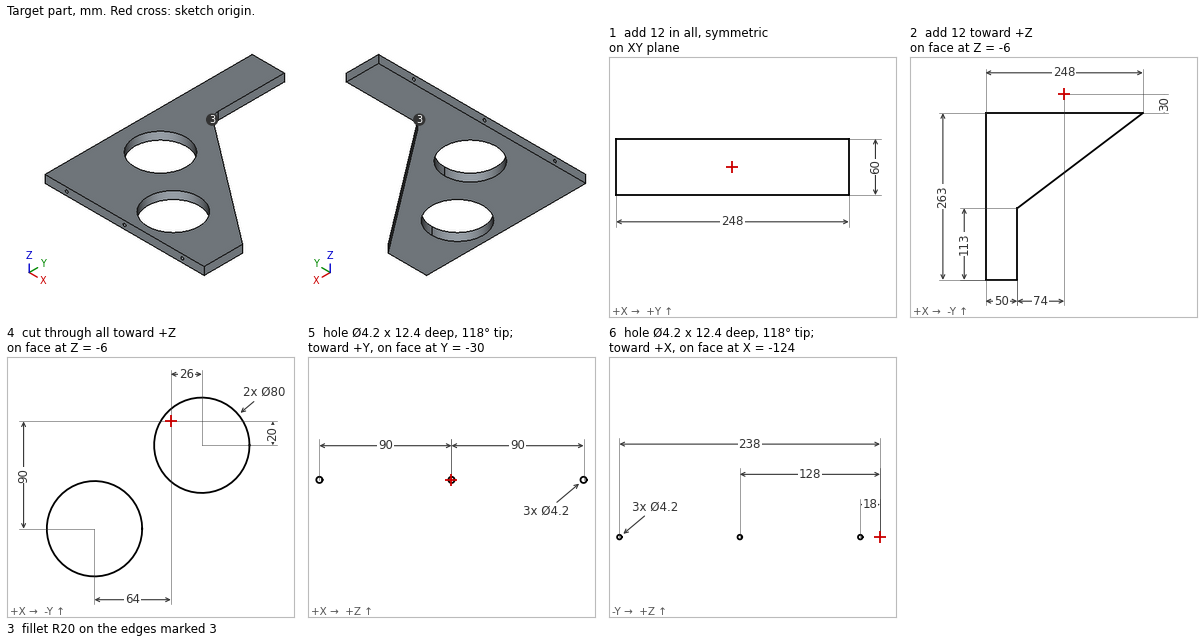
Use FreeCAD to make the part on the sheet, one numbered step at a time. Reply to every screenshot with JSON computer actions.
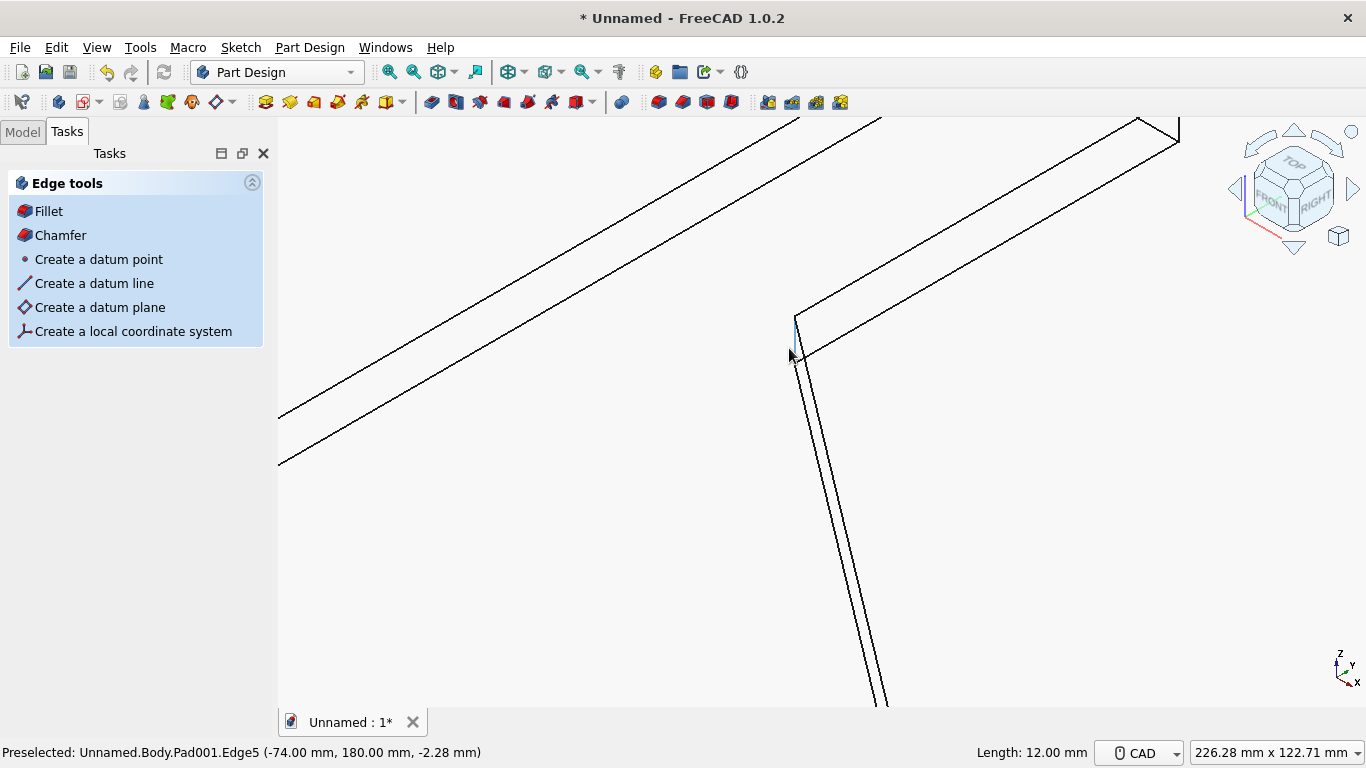
{"action": "key", "text": "v 1"}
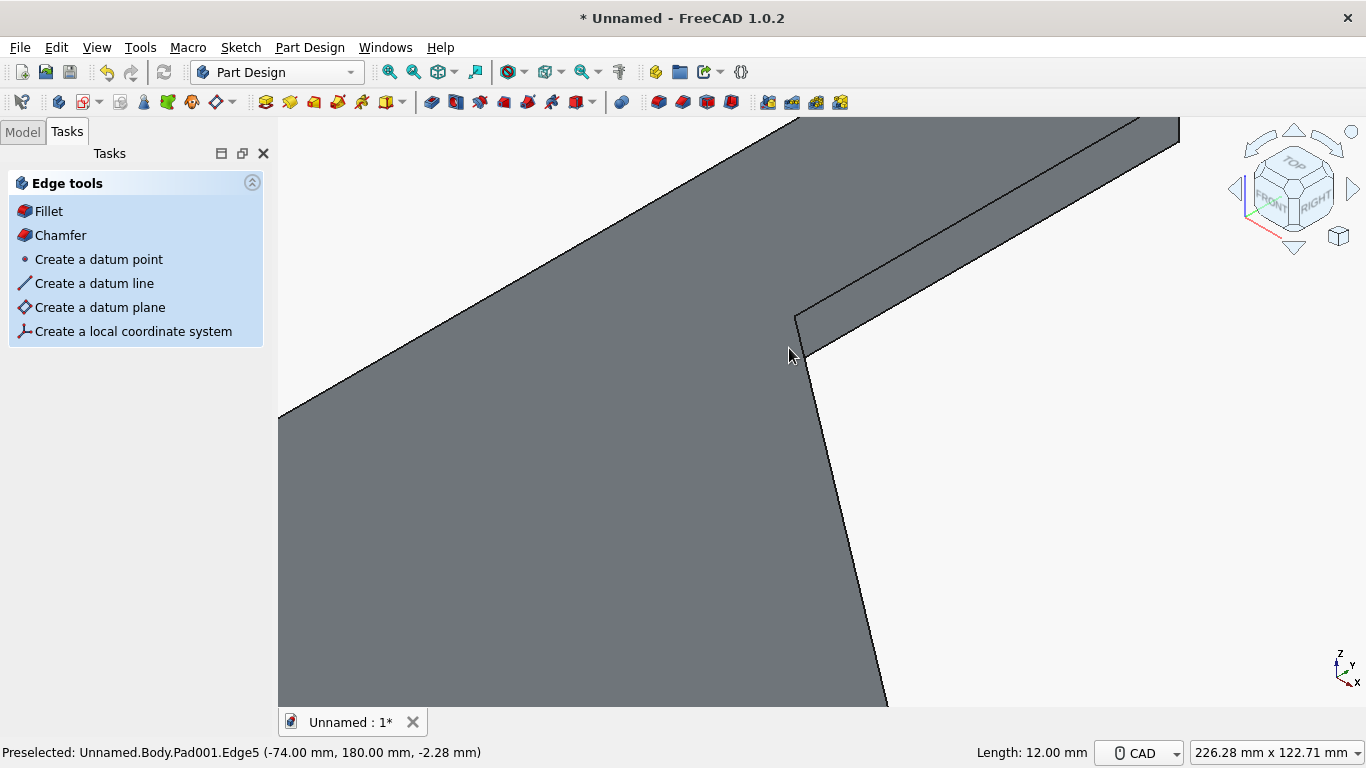
{"action": "left_click", "coordinate": [660, 102]}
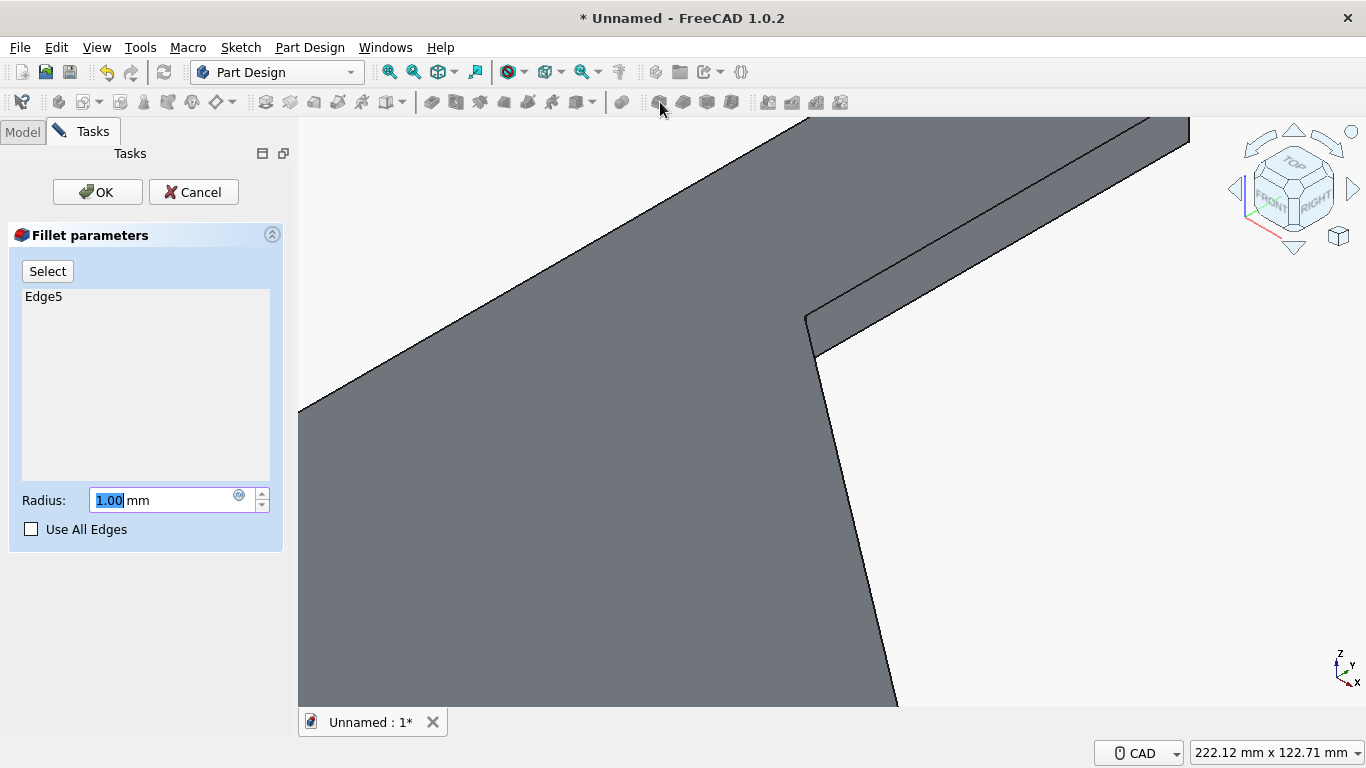
{"action": "type", "text": "20"}
{"action": "key", "text": "Tab"}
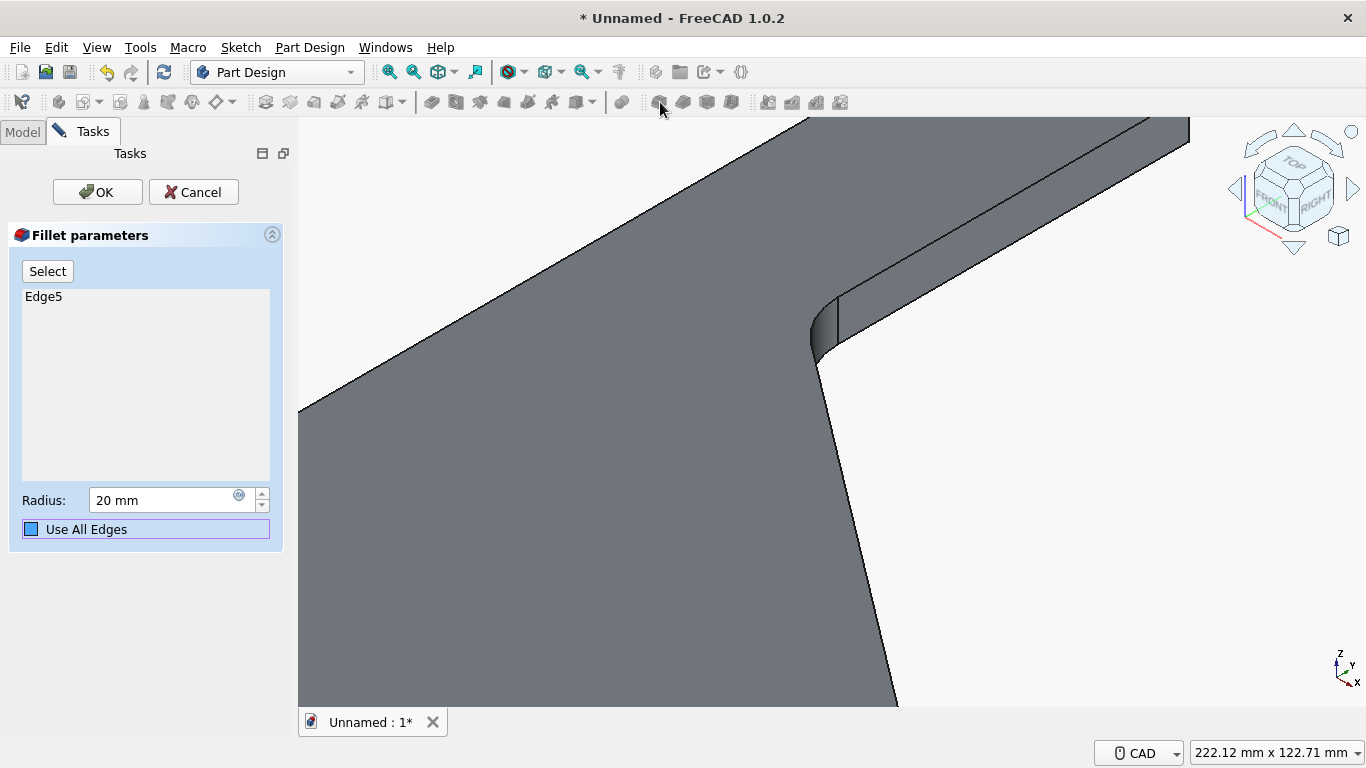
{"action": "left_click", "coordinate": [98, 192]}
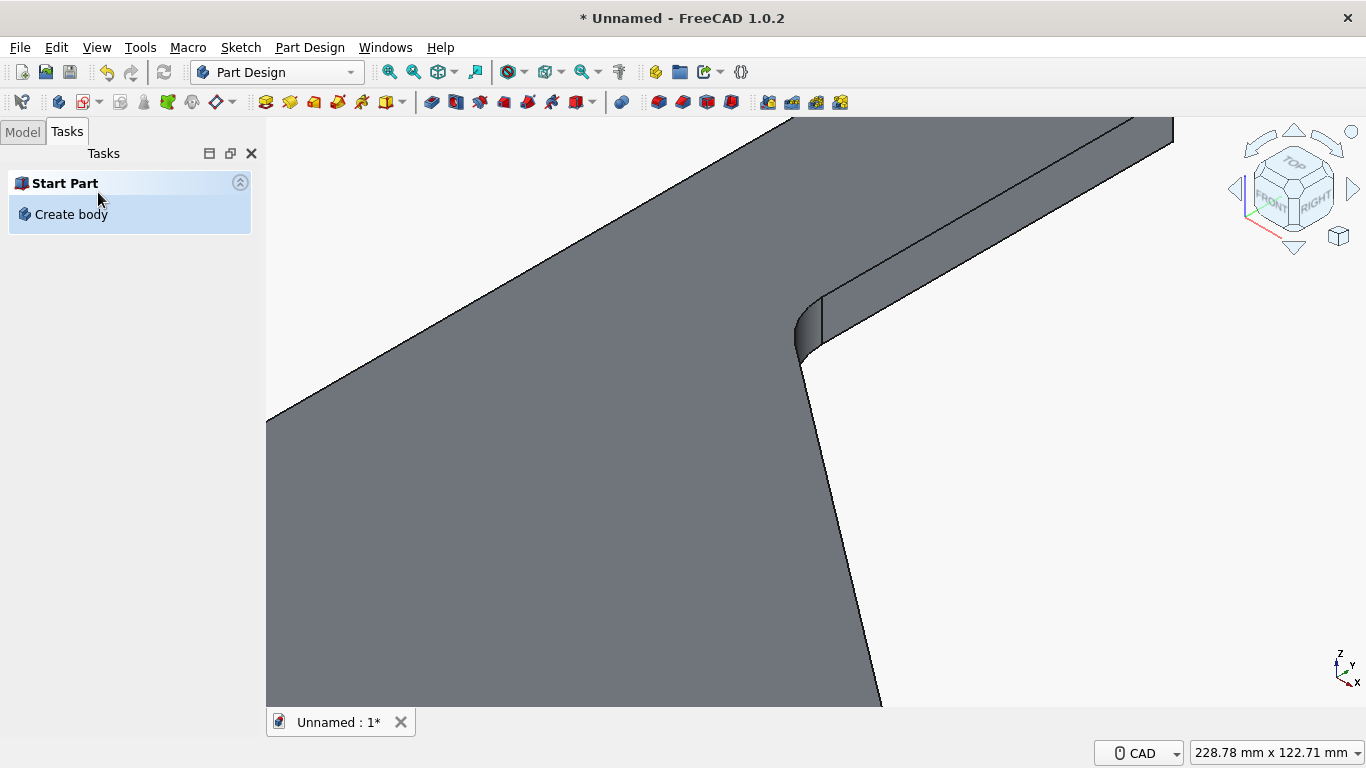
{"action": "left_click", "coordinate": [390, 72]}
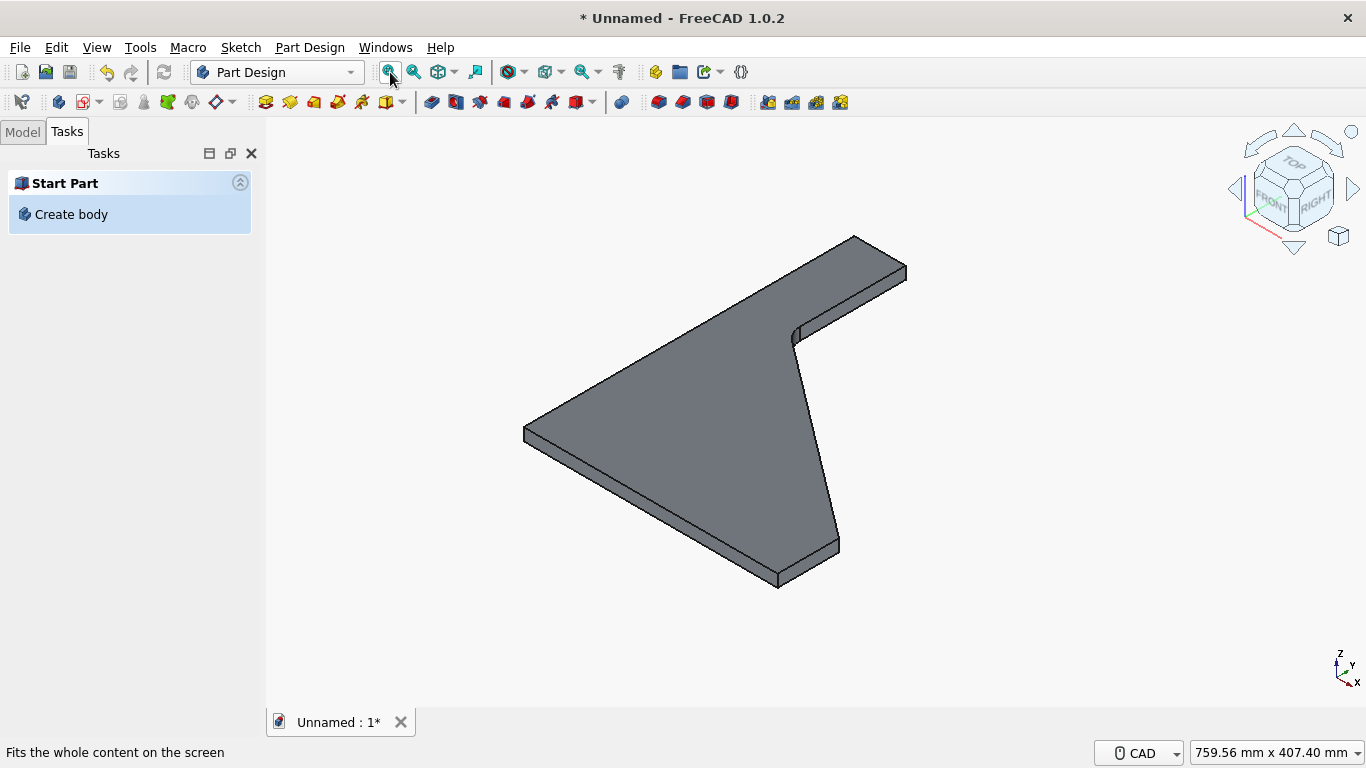
{"action": "key", "text": "5"}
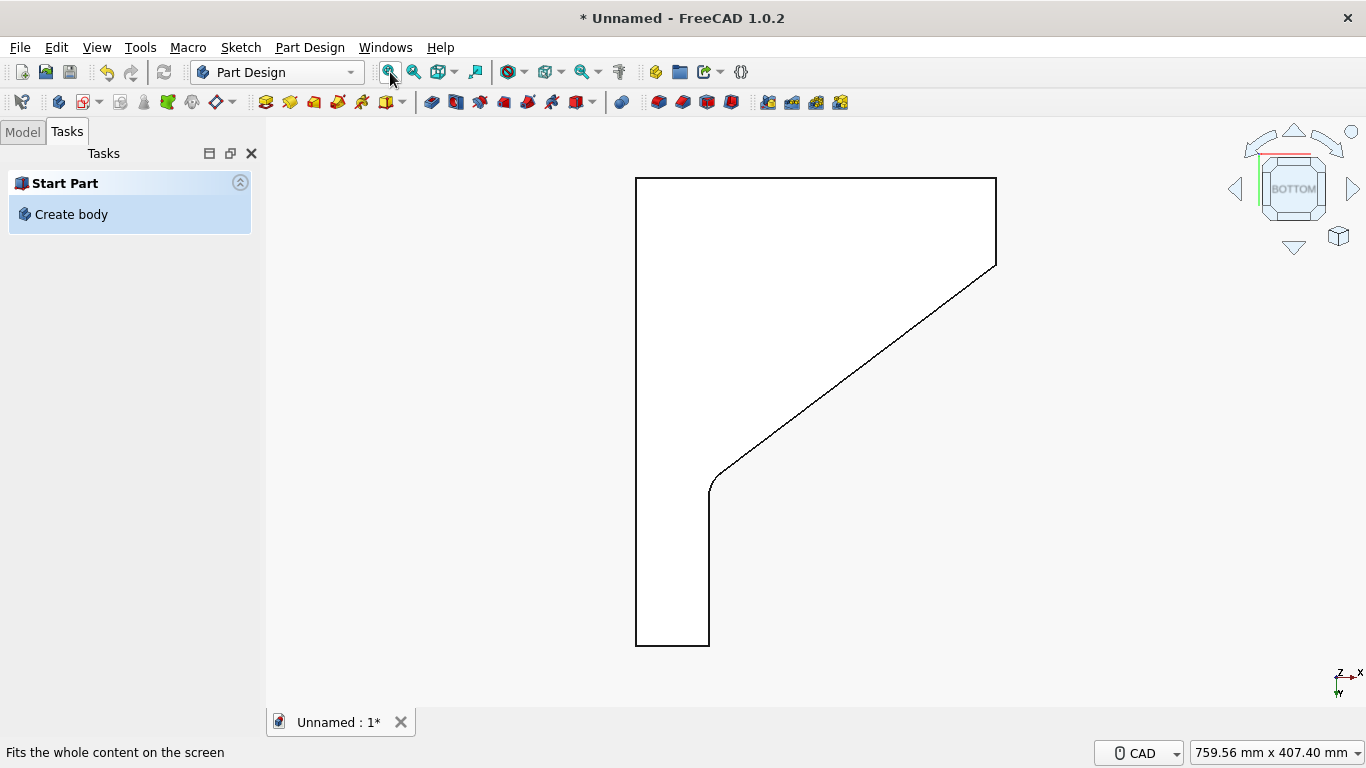
{"action": "left_click", "coordinate": [765, 277]}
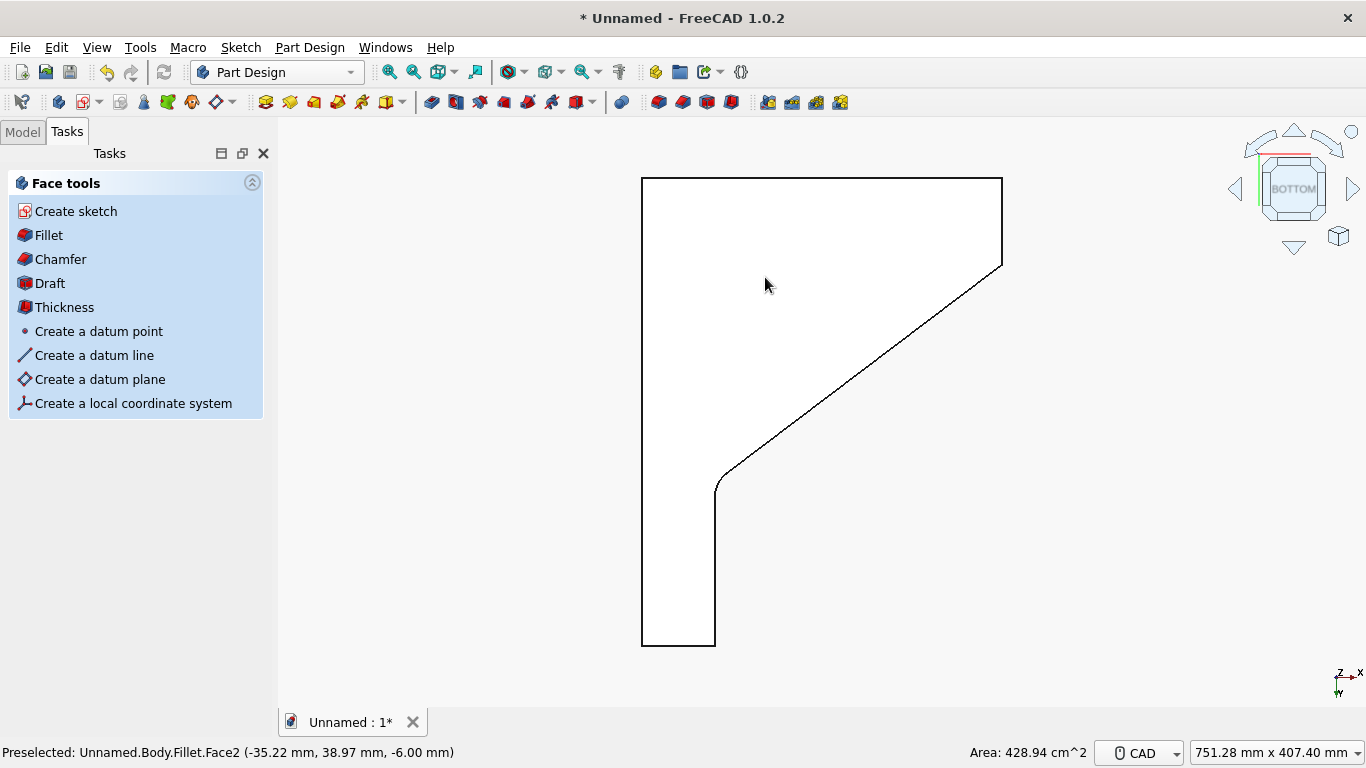
{"action": "left_click", "coordinate": [84, 102]}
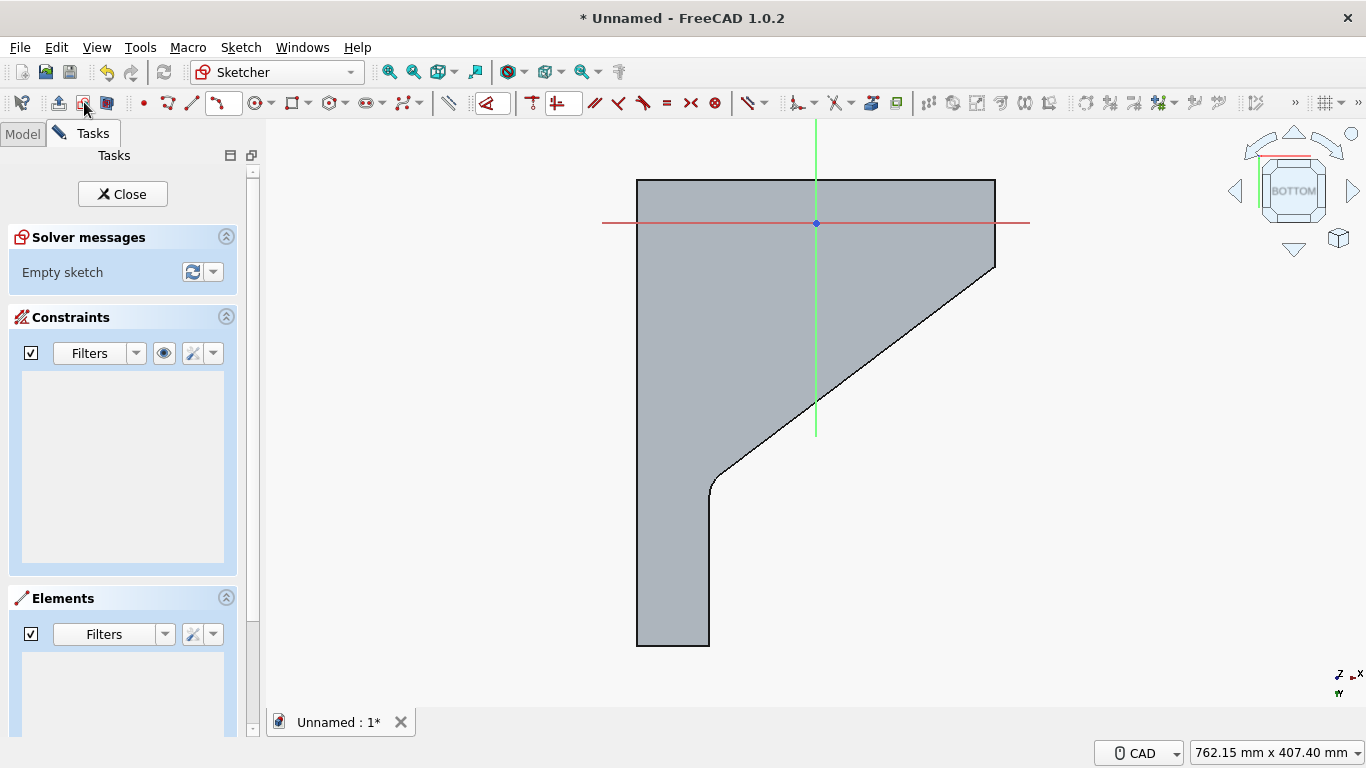
{"action": "scroll", "coordinate": [839, 168], "scroll_direction": "up", "scroll_amount": 3}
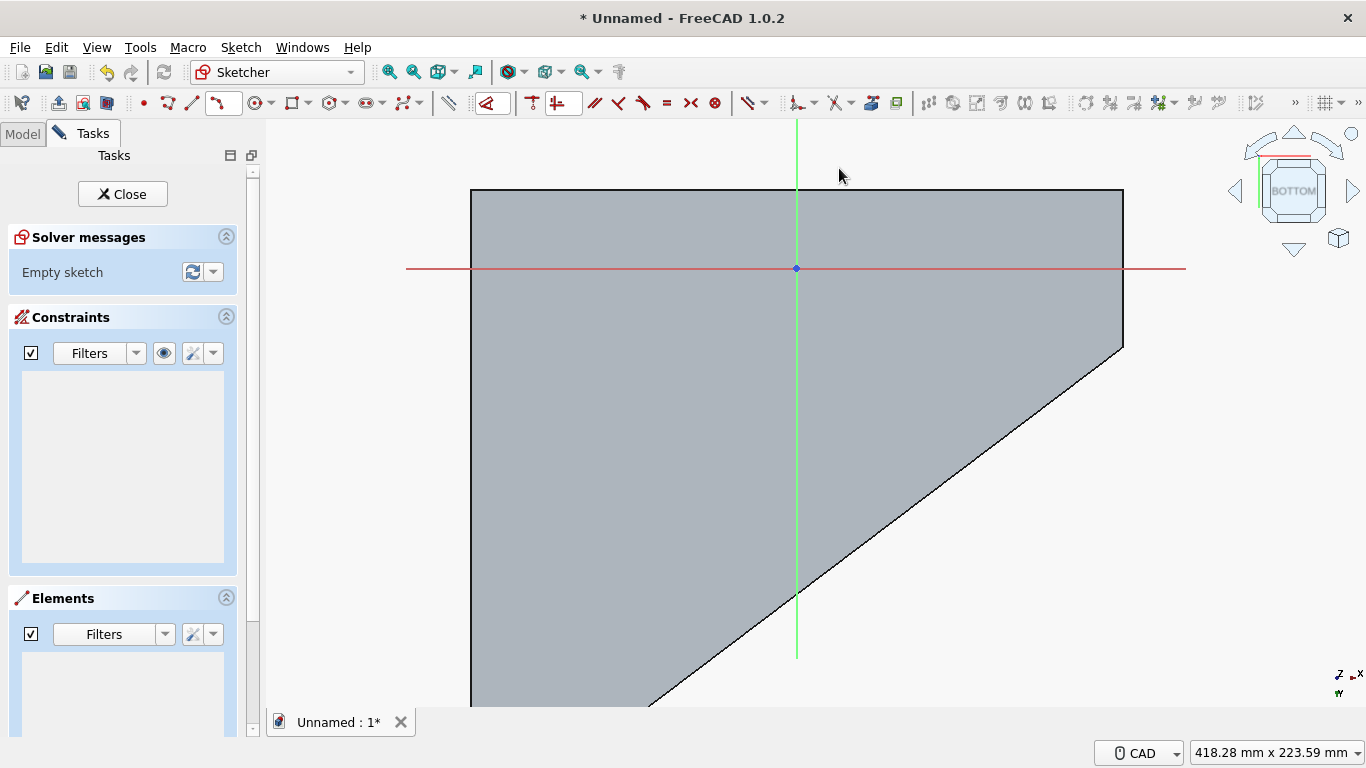
{"action": "key", "text": "g c"}